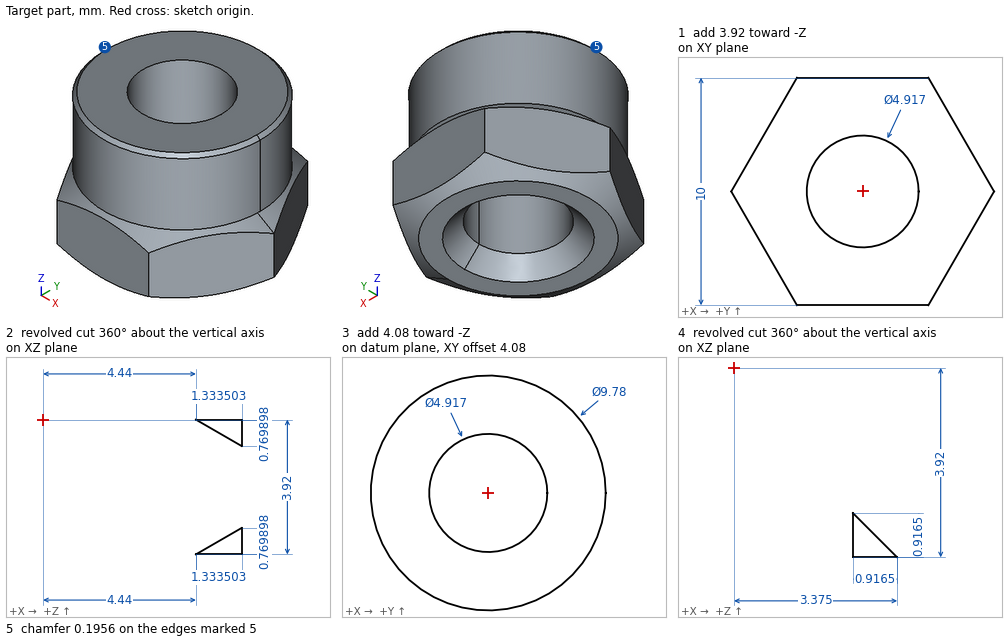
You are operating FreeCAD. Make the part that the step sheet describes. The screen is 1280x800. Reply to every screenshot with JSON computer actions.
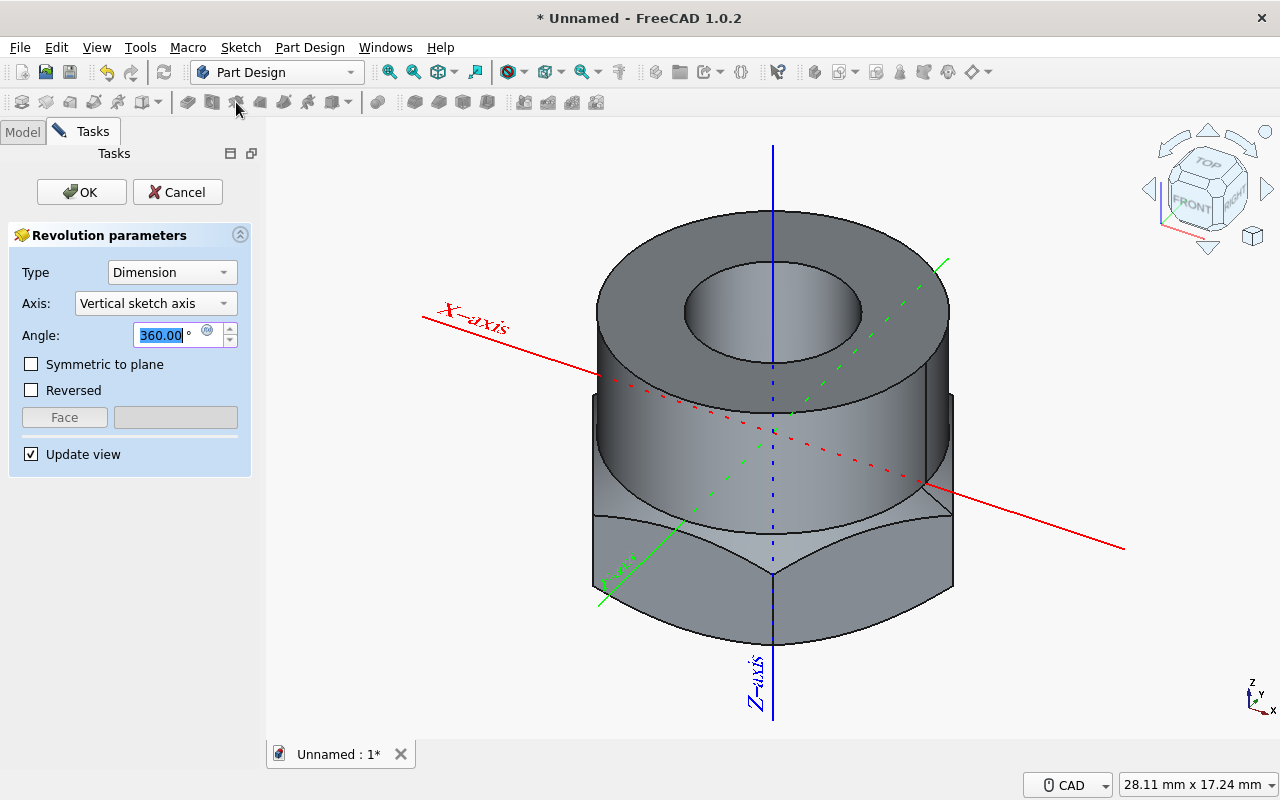
{"action": "left_click", "coordinate": [82, 192]}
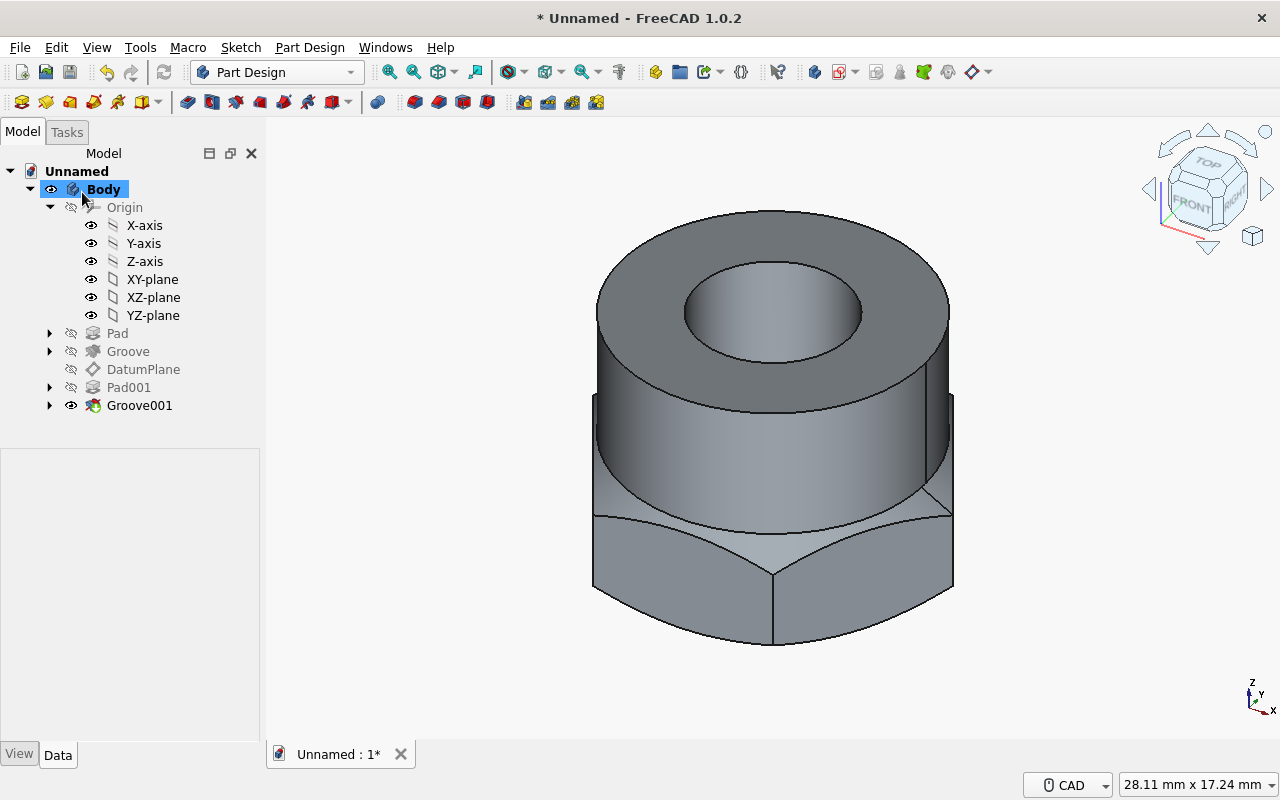
{"action": "left_click", "coordinate": [598, 322]}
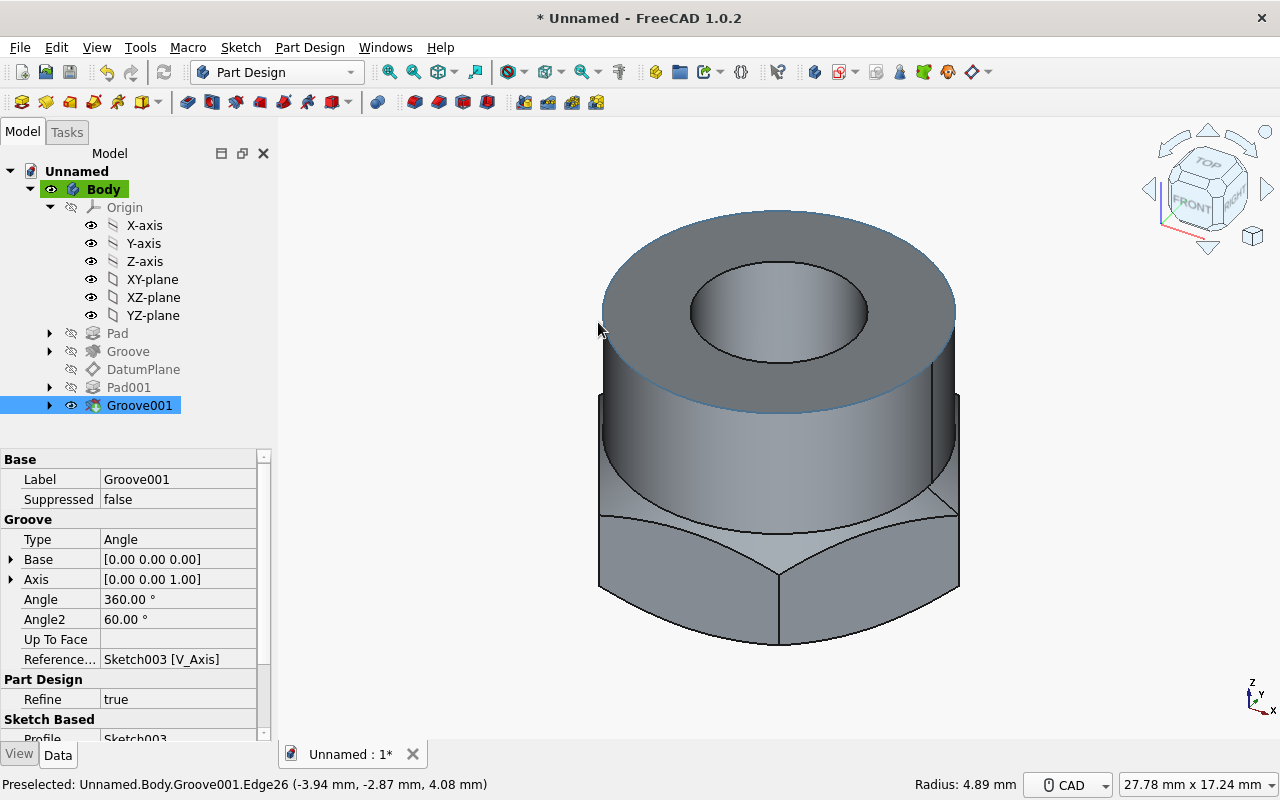
{"action": "left_click", "coordinate": [440, 102]}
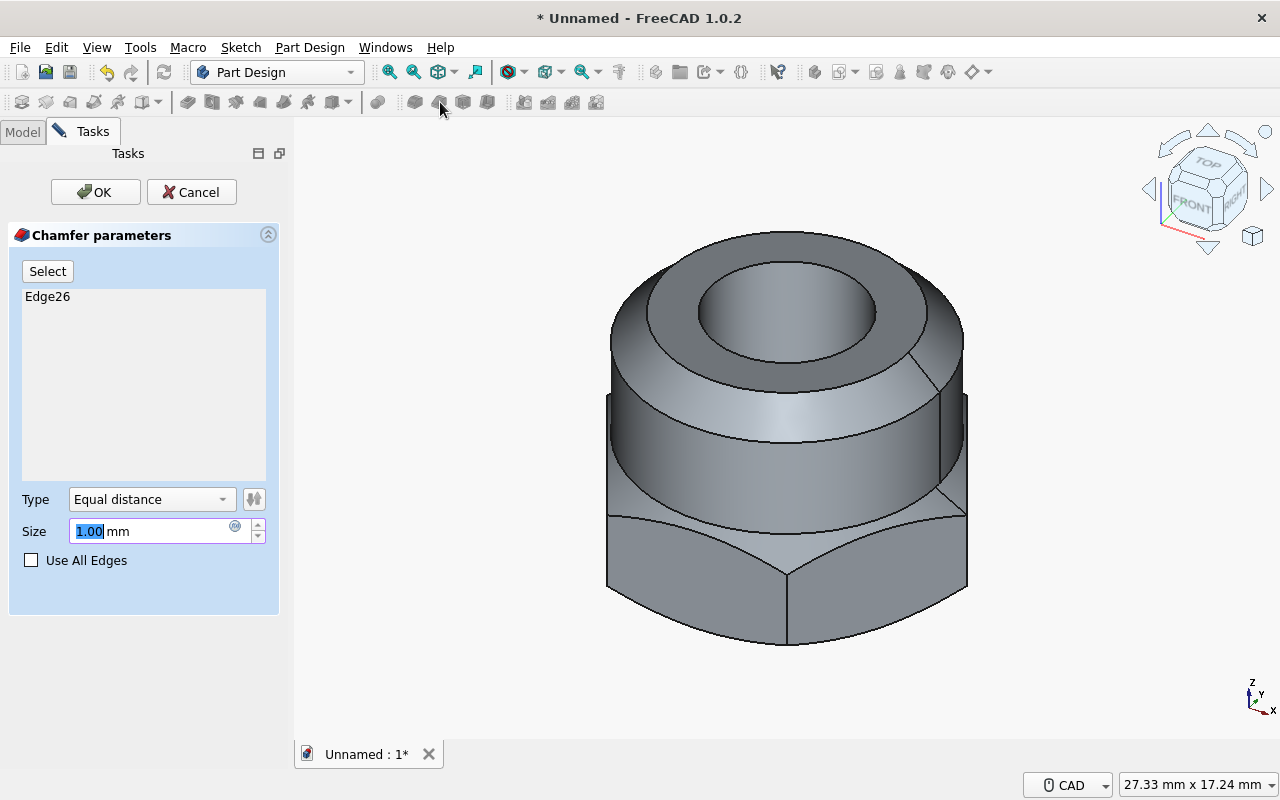
{"action": "type", "text": "0.1956"}
{"action": "key", "text": "Tab"}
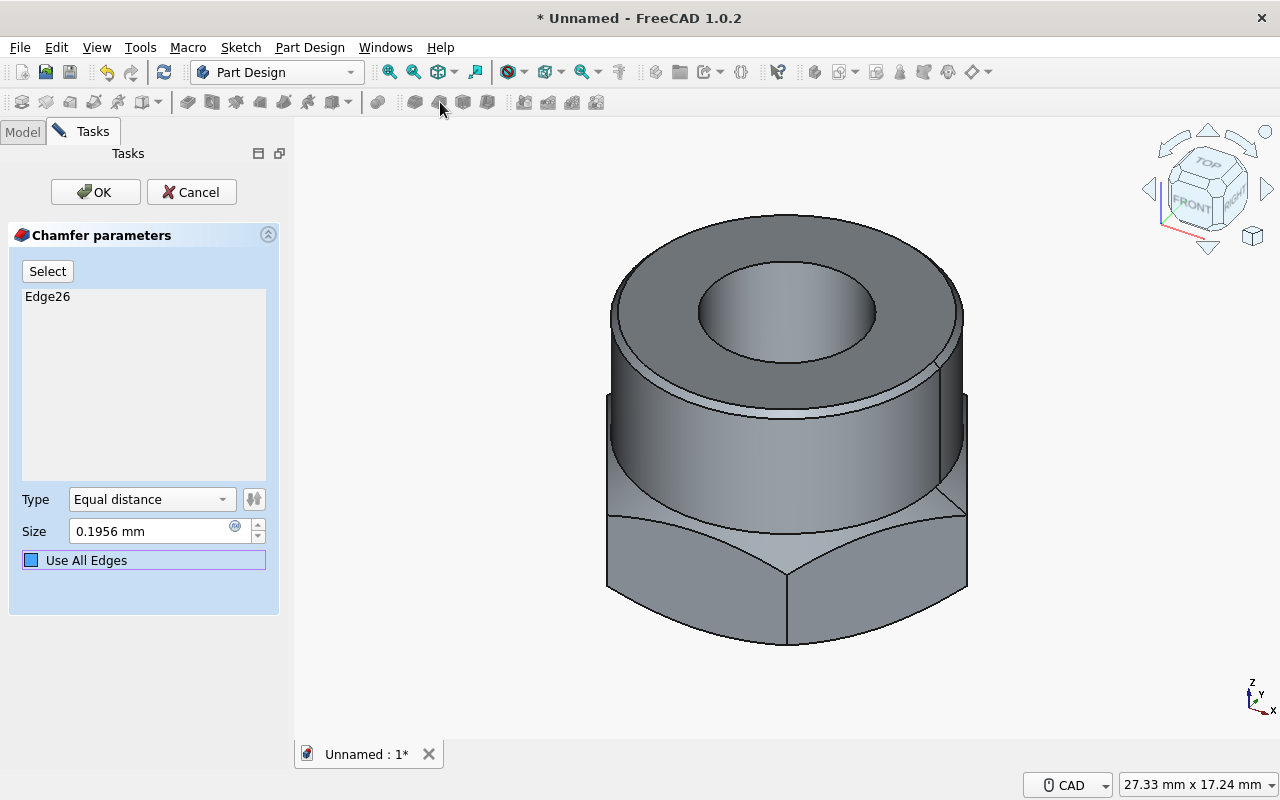
{"action": "left_click", "coordinate": [96, 192]}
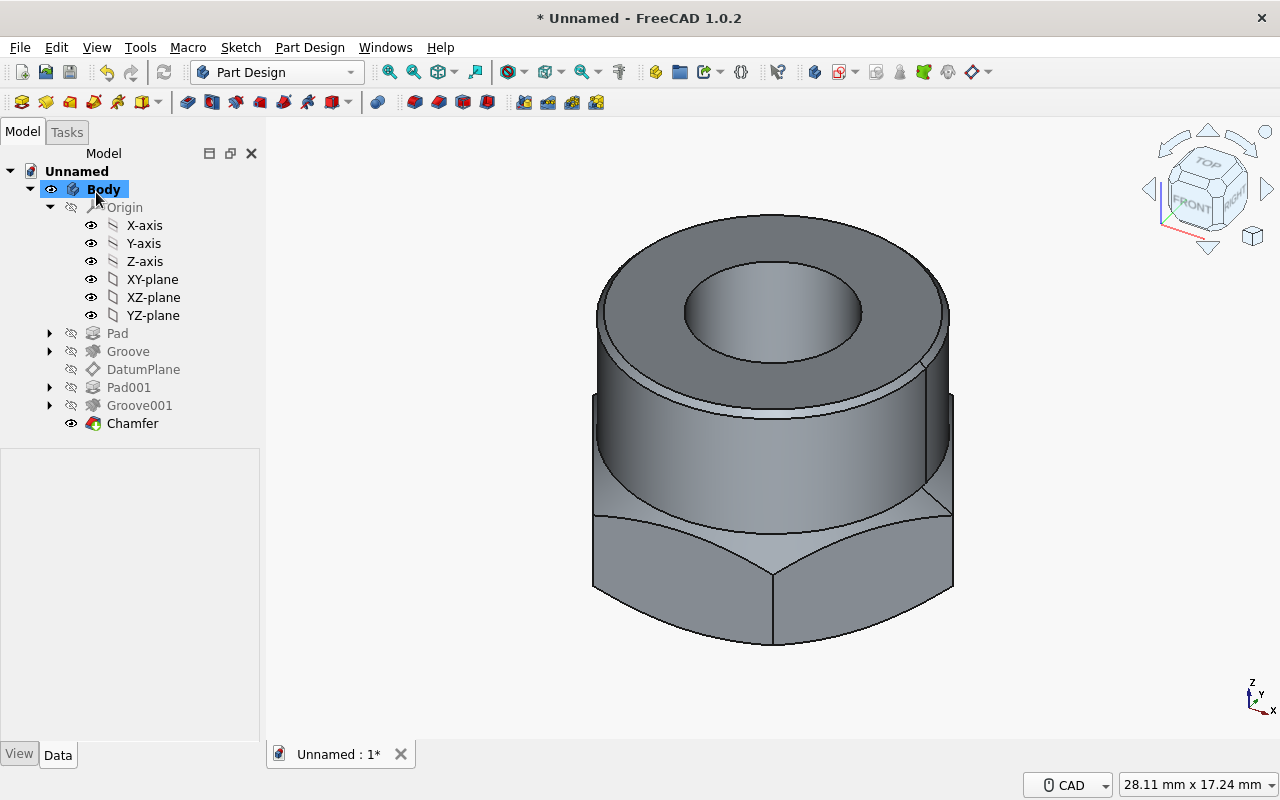
{"action": "key", "text": "0"}